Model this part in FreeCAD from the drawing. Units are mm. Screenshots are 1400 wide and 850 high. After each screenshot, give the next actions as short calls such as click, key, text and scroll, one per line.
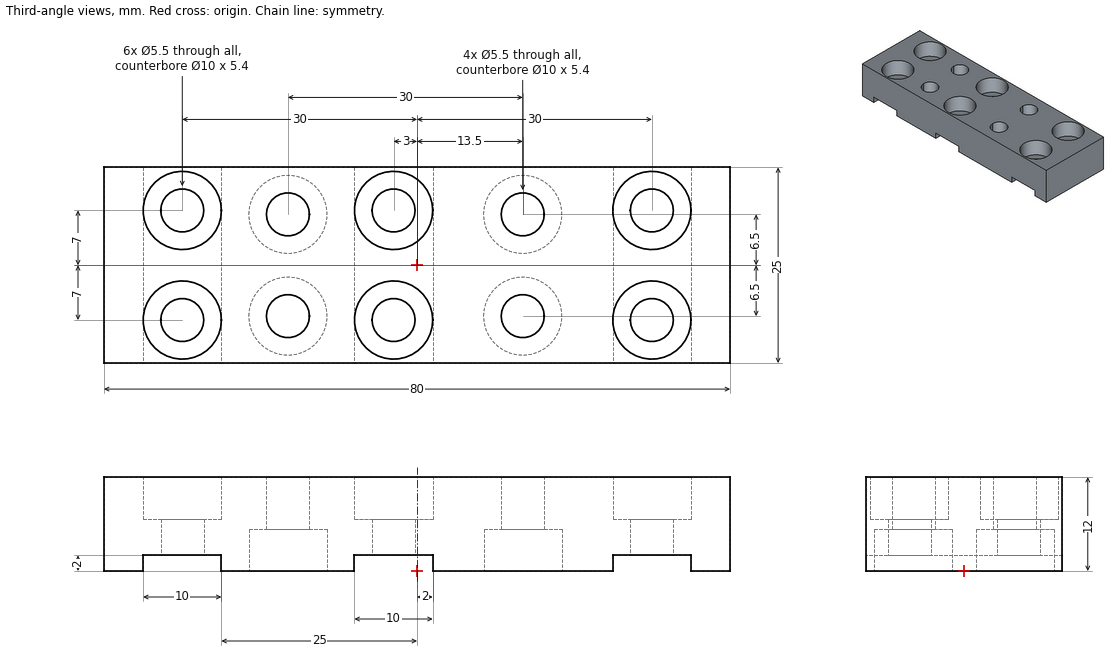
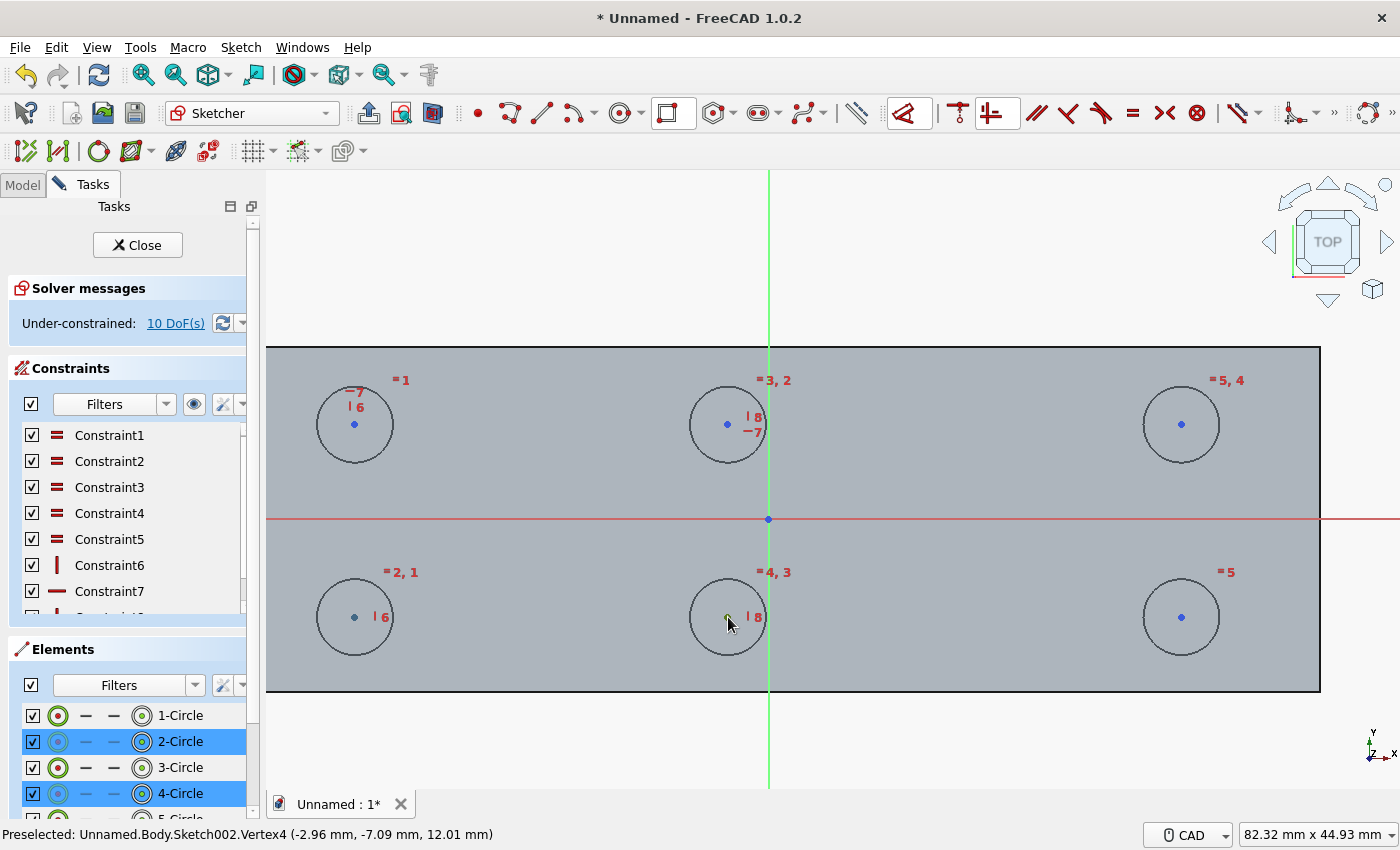
click(1014, 114)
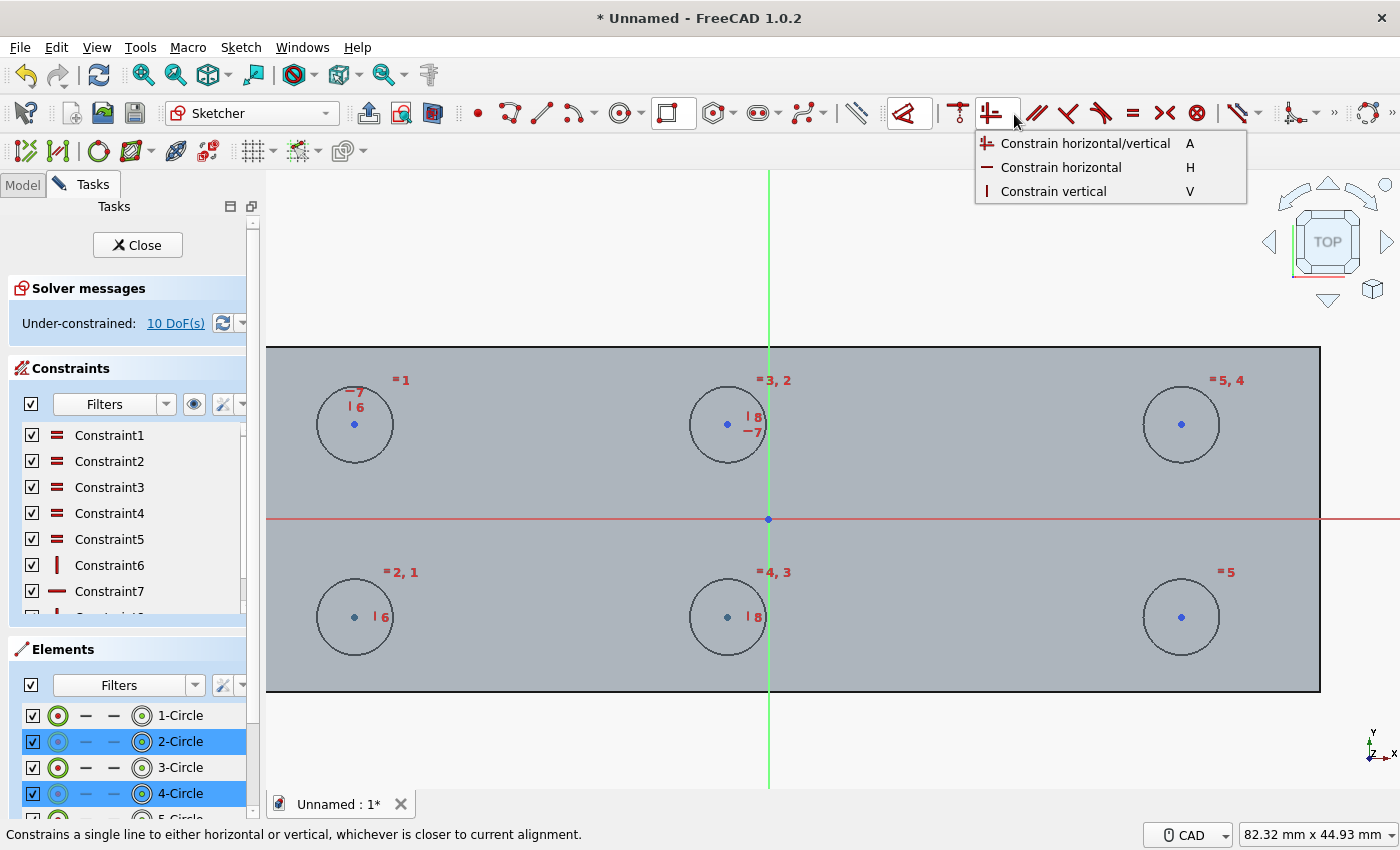
click(1111, 167)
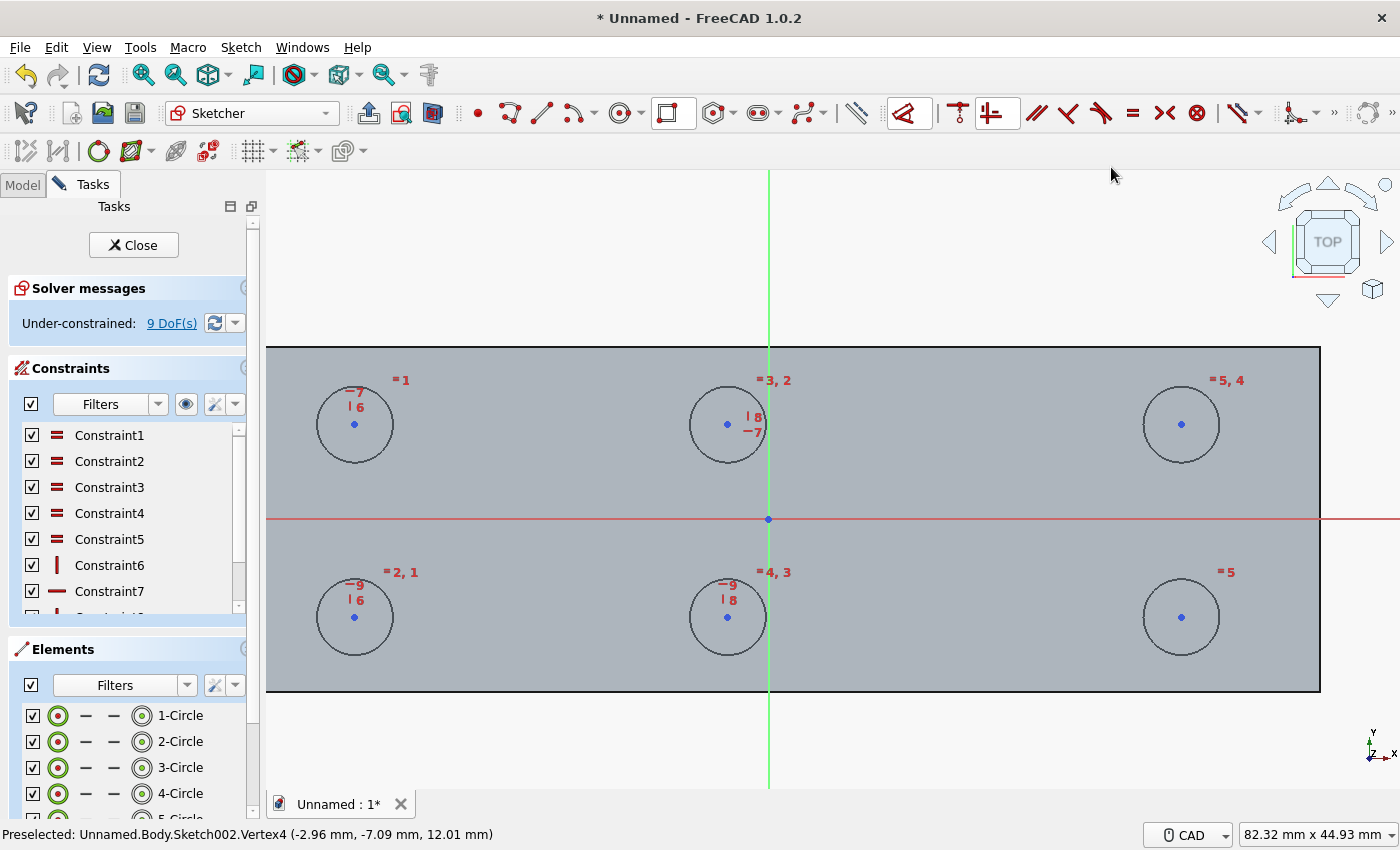
click(728, 425)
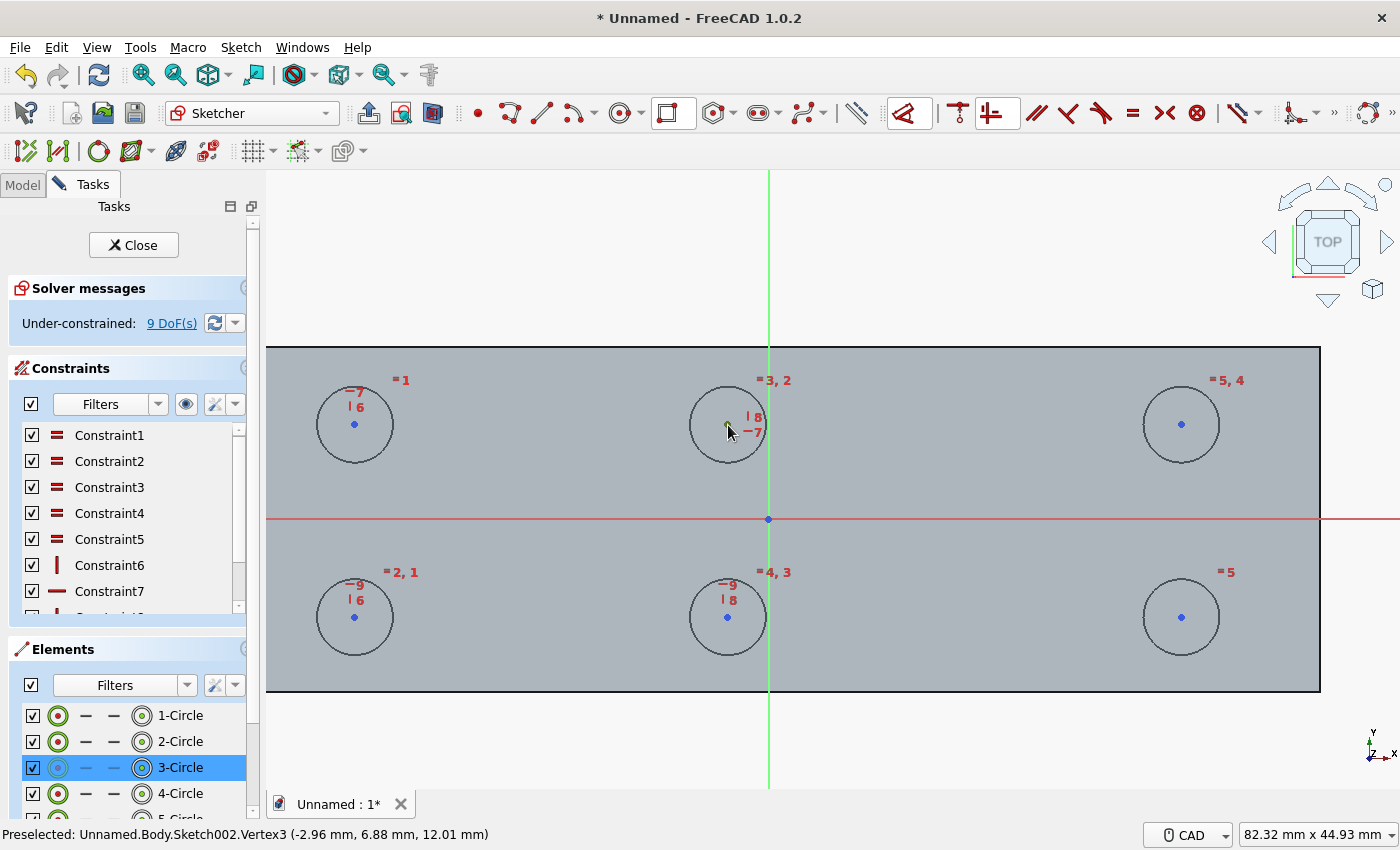
click(1181, 425)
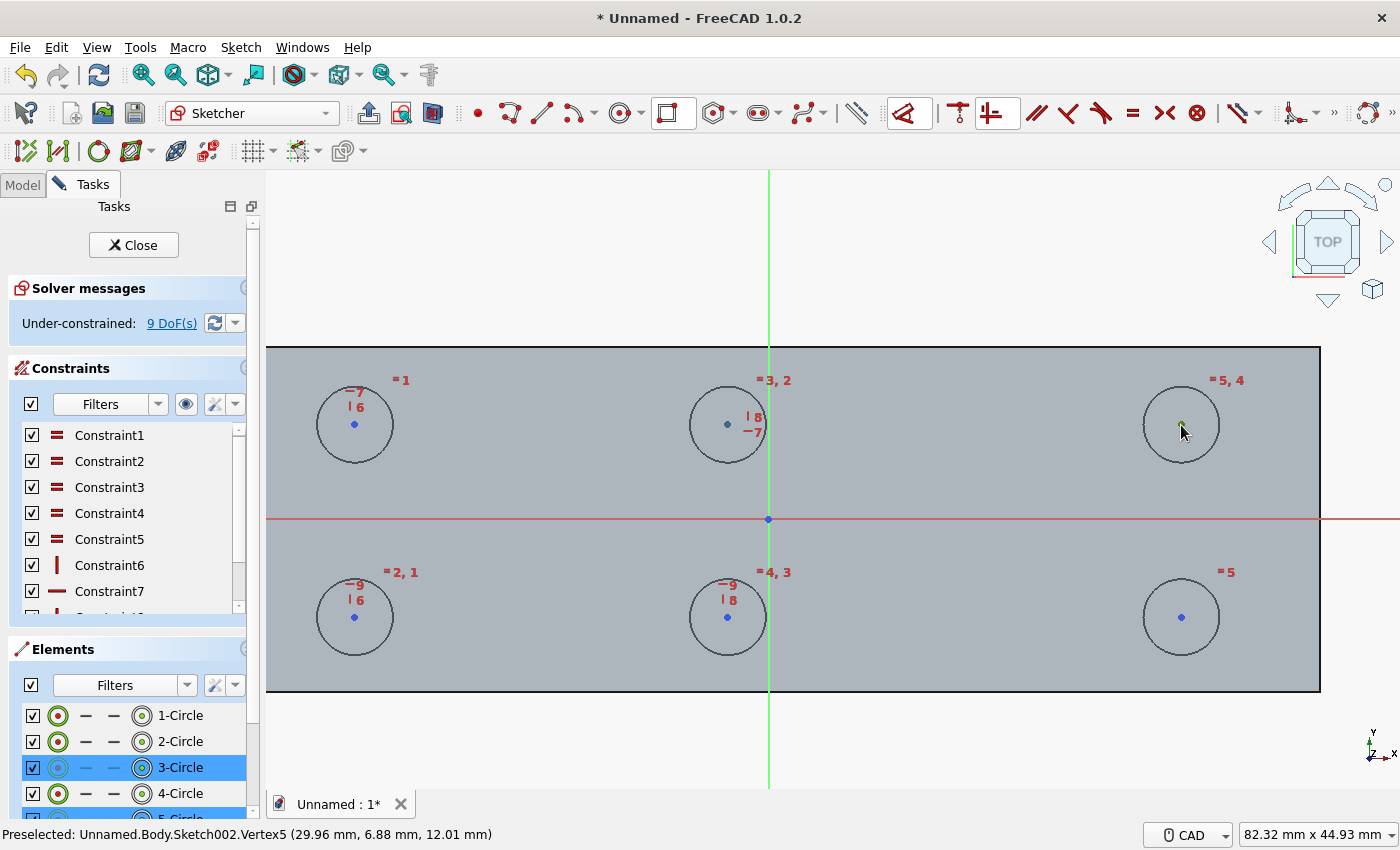
key(h)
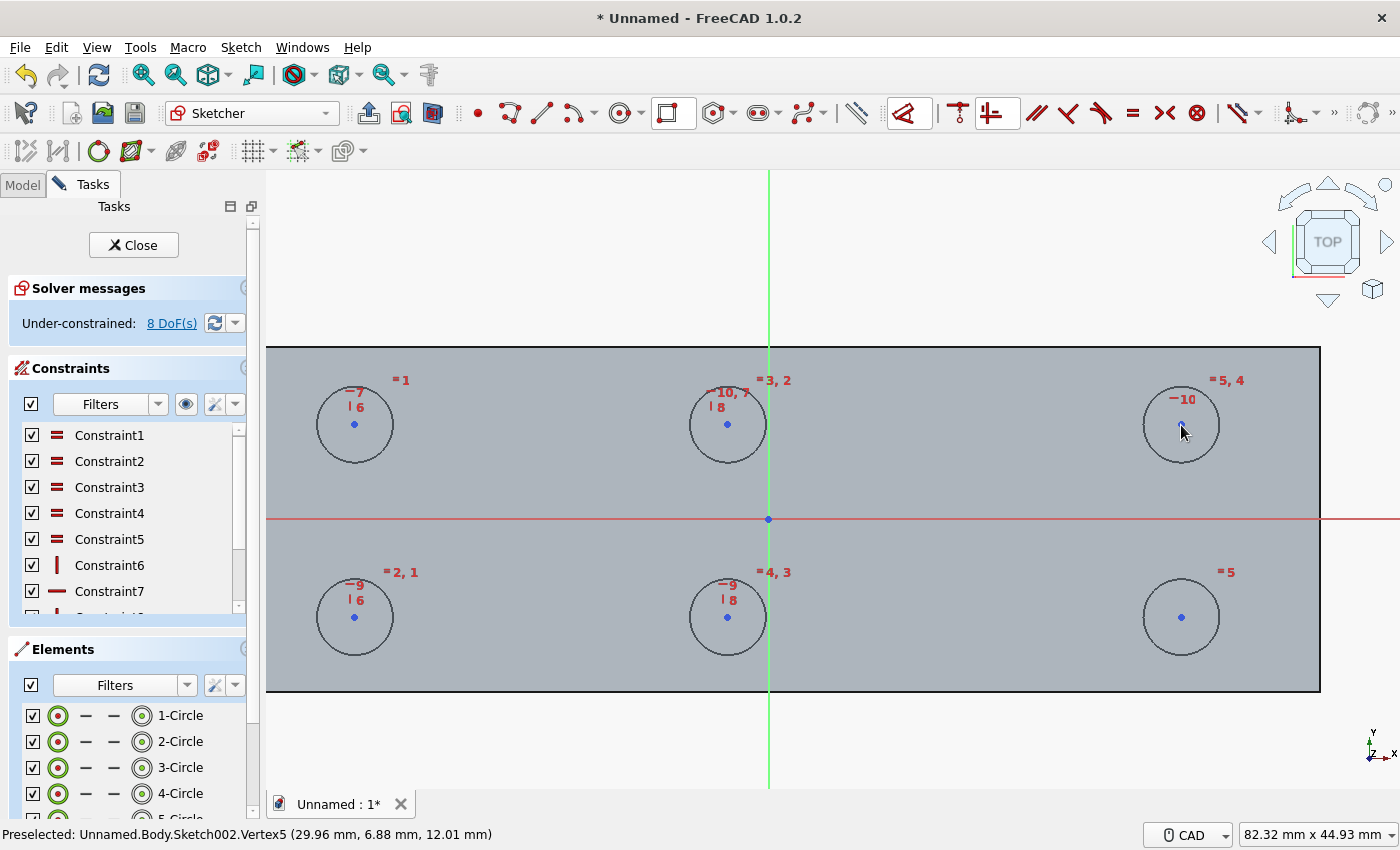
click(1181, 425)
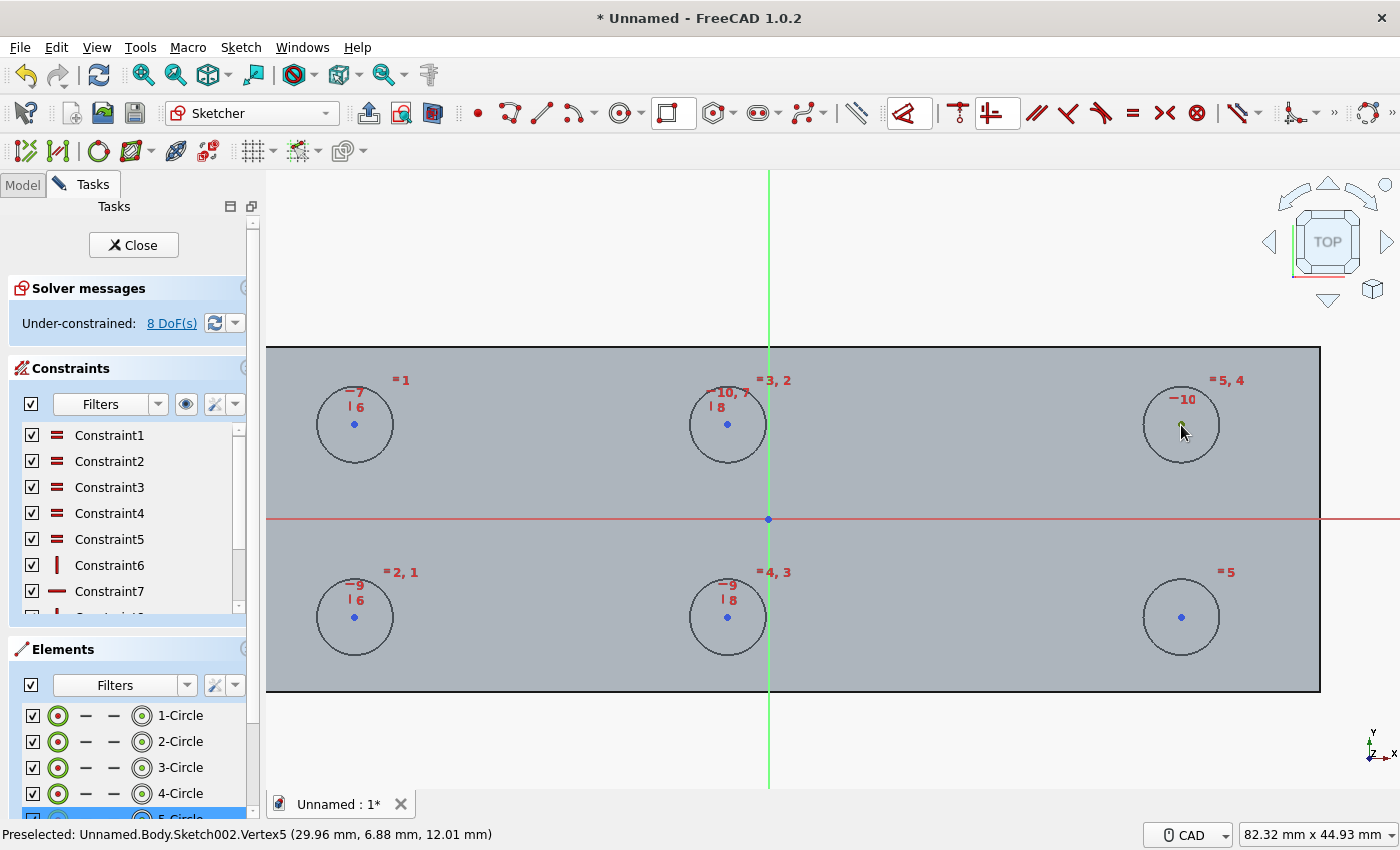
click(1181, 617)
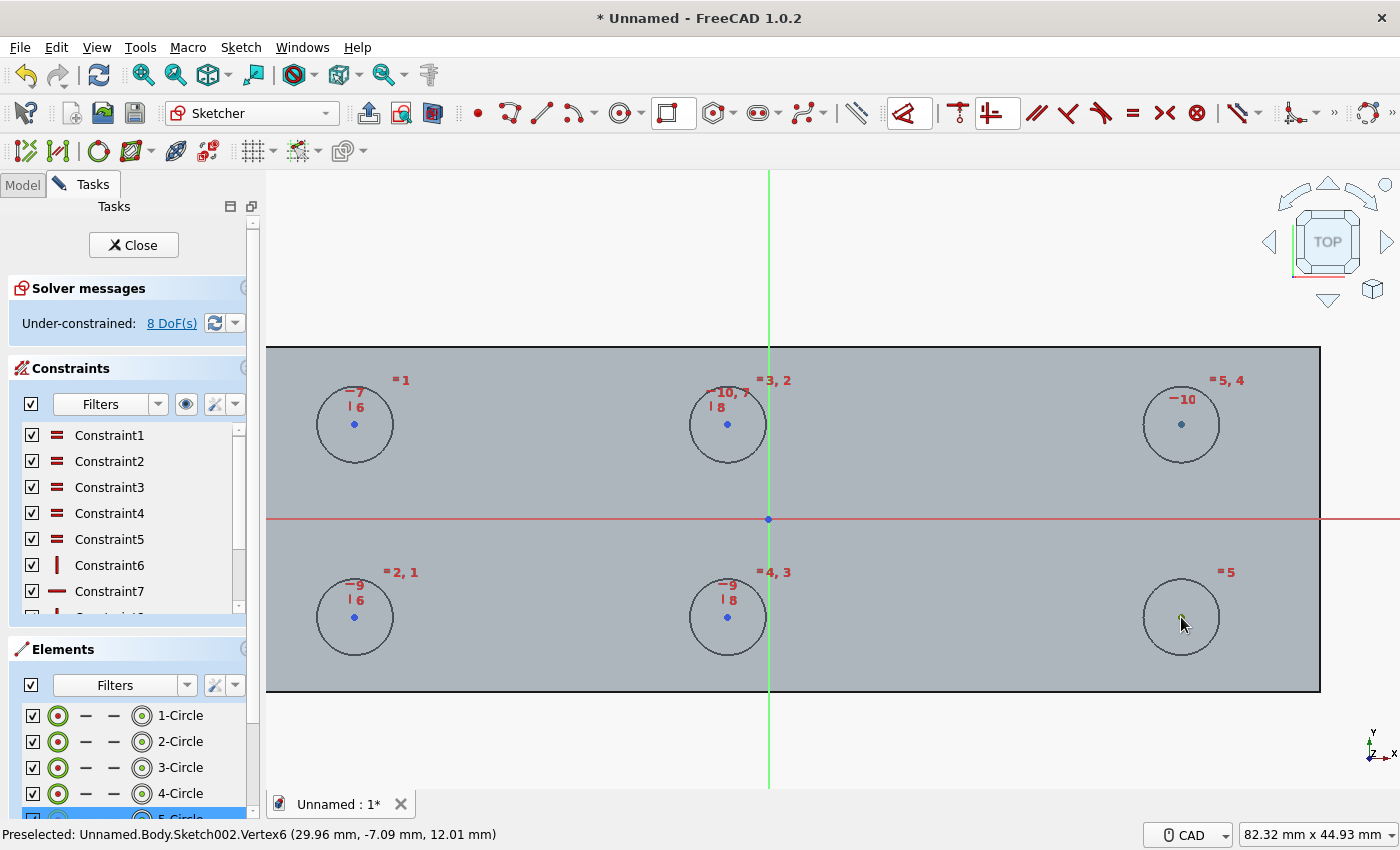
key(v)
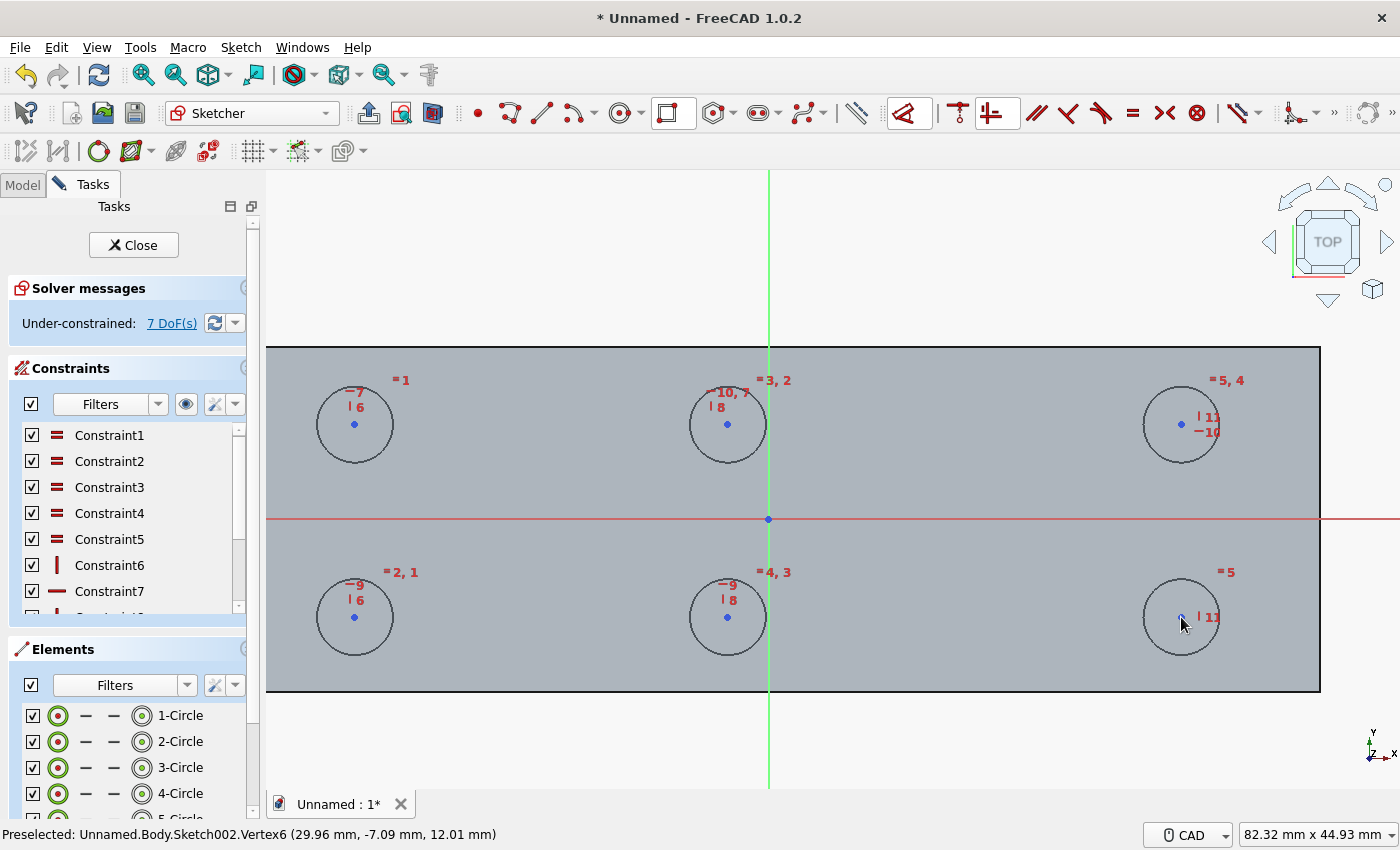
click(728, 617)